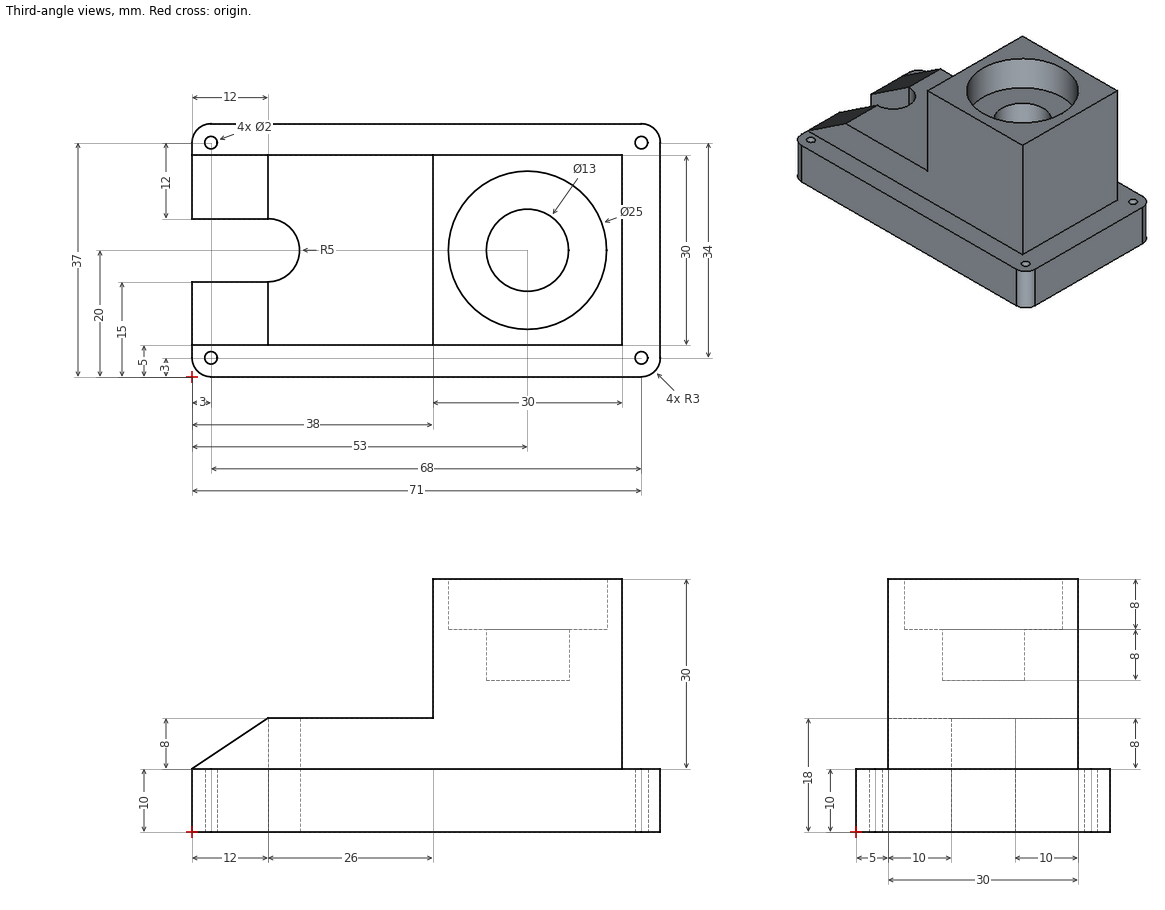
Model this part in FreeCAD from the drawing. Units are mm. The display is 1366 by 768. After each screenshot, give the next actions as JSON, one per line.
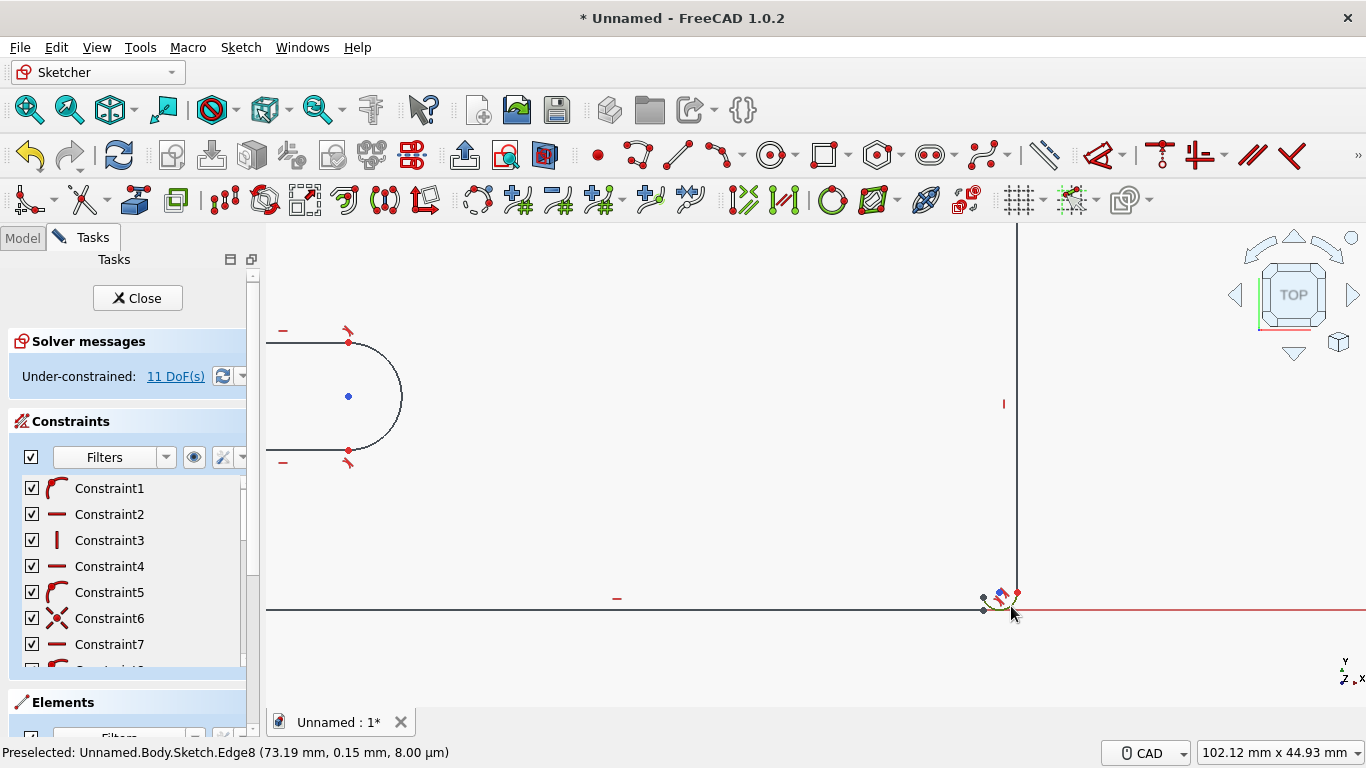
{"action": "scroll", "coordinate": [1013, 608], "scroll_direction": "down", "scroll_amount": 2}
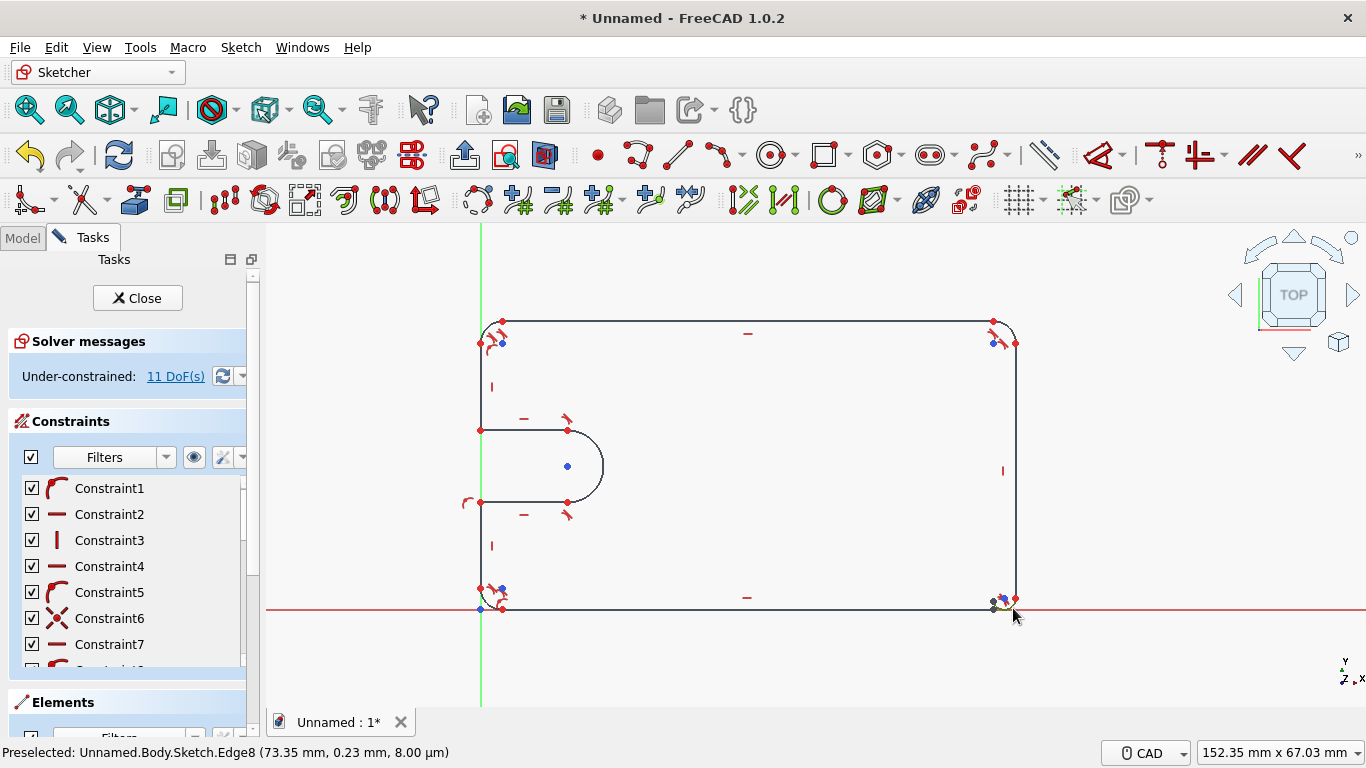
{"action": "scroll", "coordinate": [1013, 334], "scroll_direction": "up", "scroll_amount": 2}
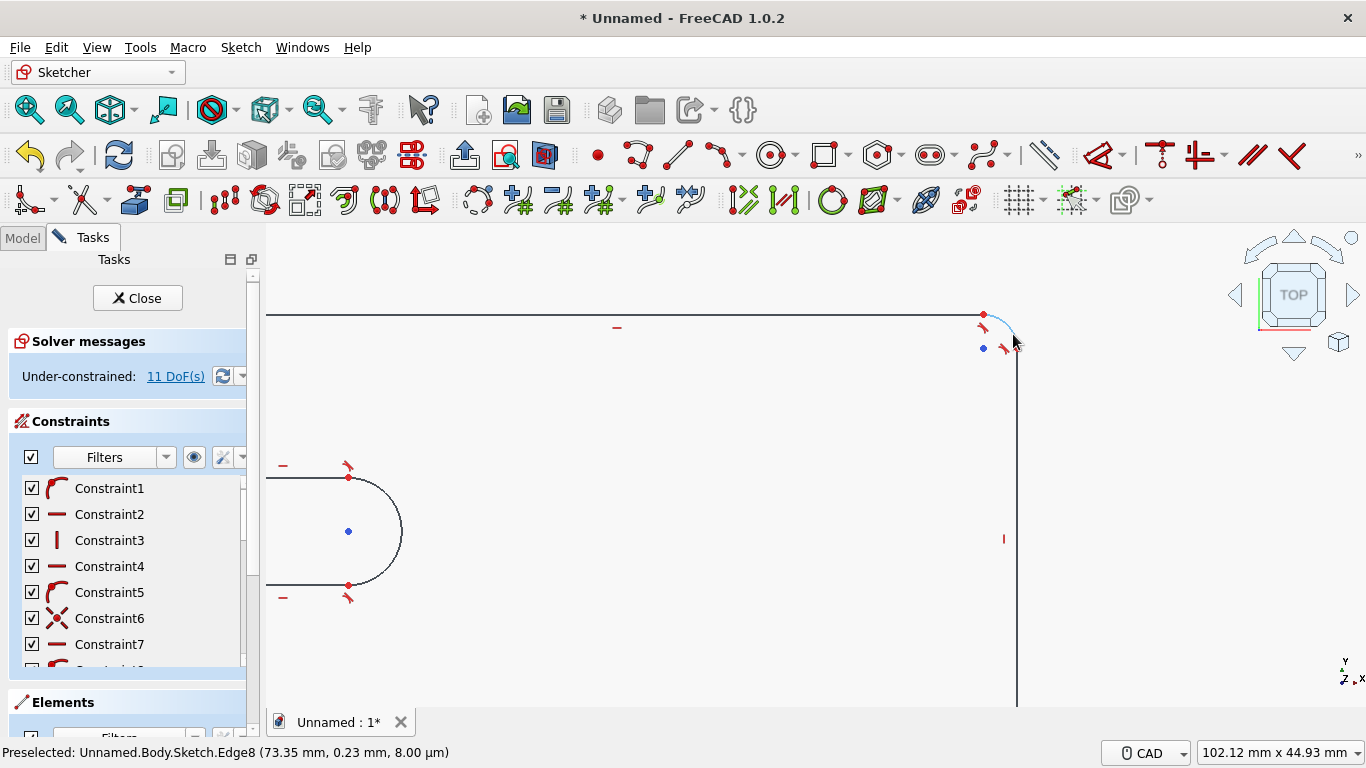
{"action": "left_click", "coordinate": [1013, 333]}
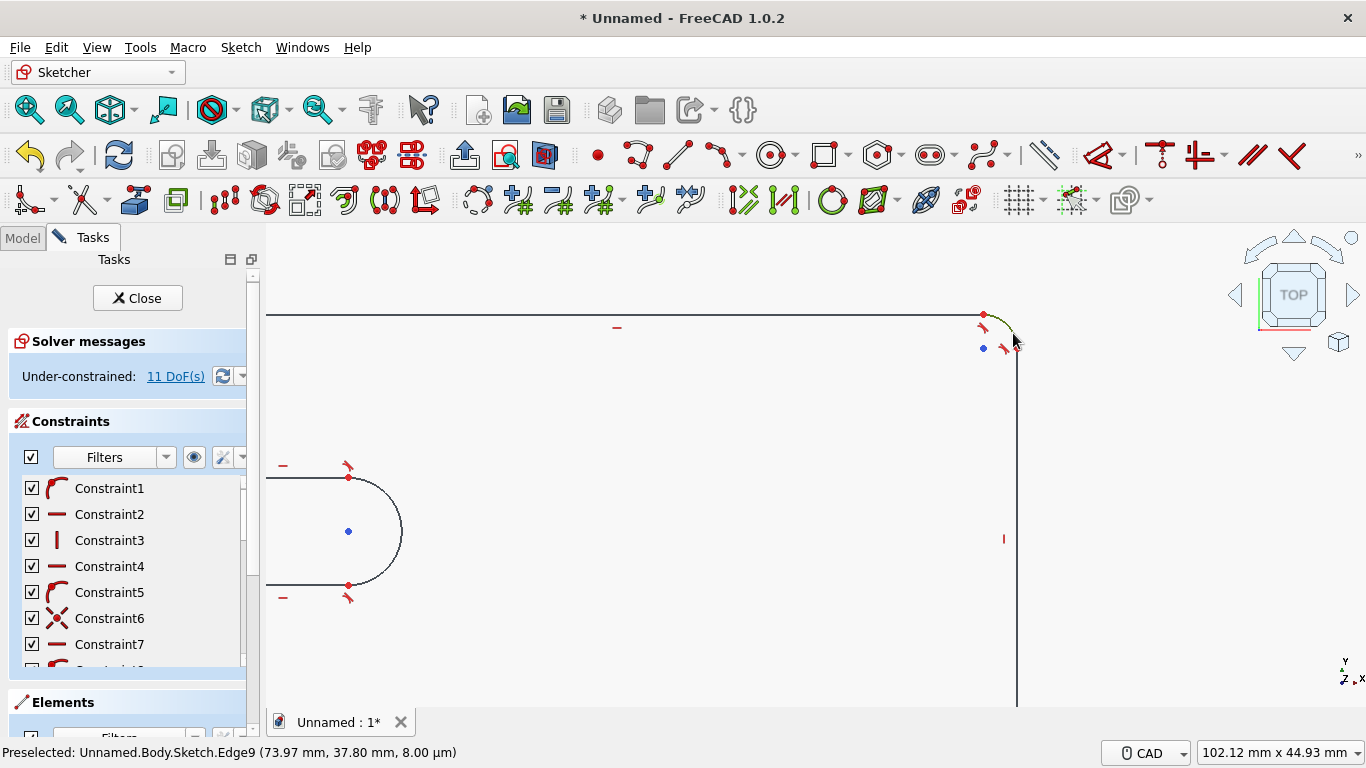
{"action": "scroll", "coordinate": [1013, 333], "scroll_direction": "down", "scroll_amount": 2}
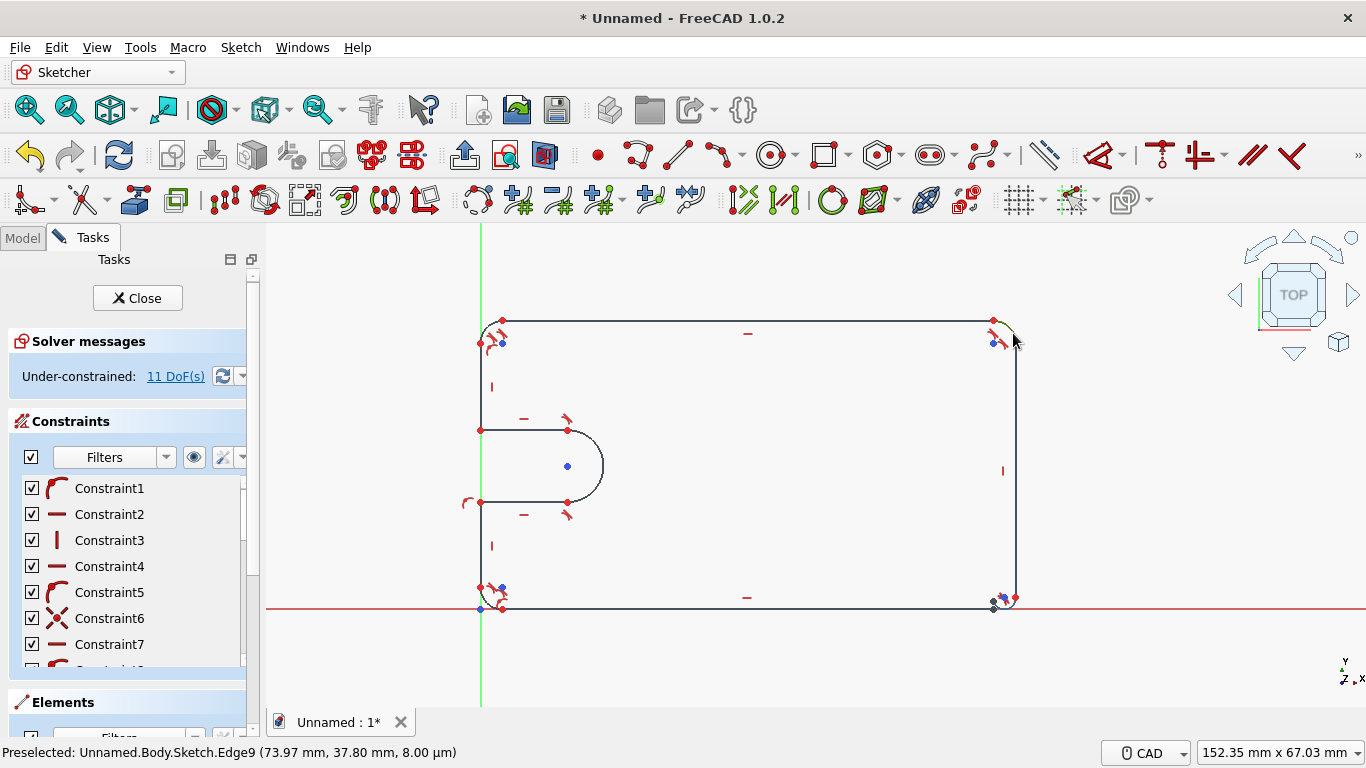
{"action": "scroll", "coordinate": [493, 323], "scroll_direction": "up", "scroll_amount": 2}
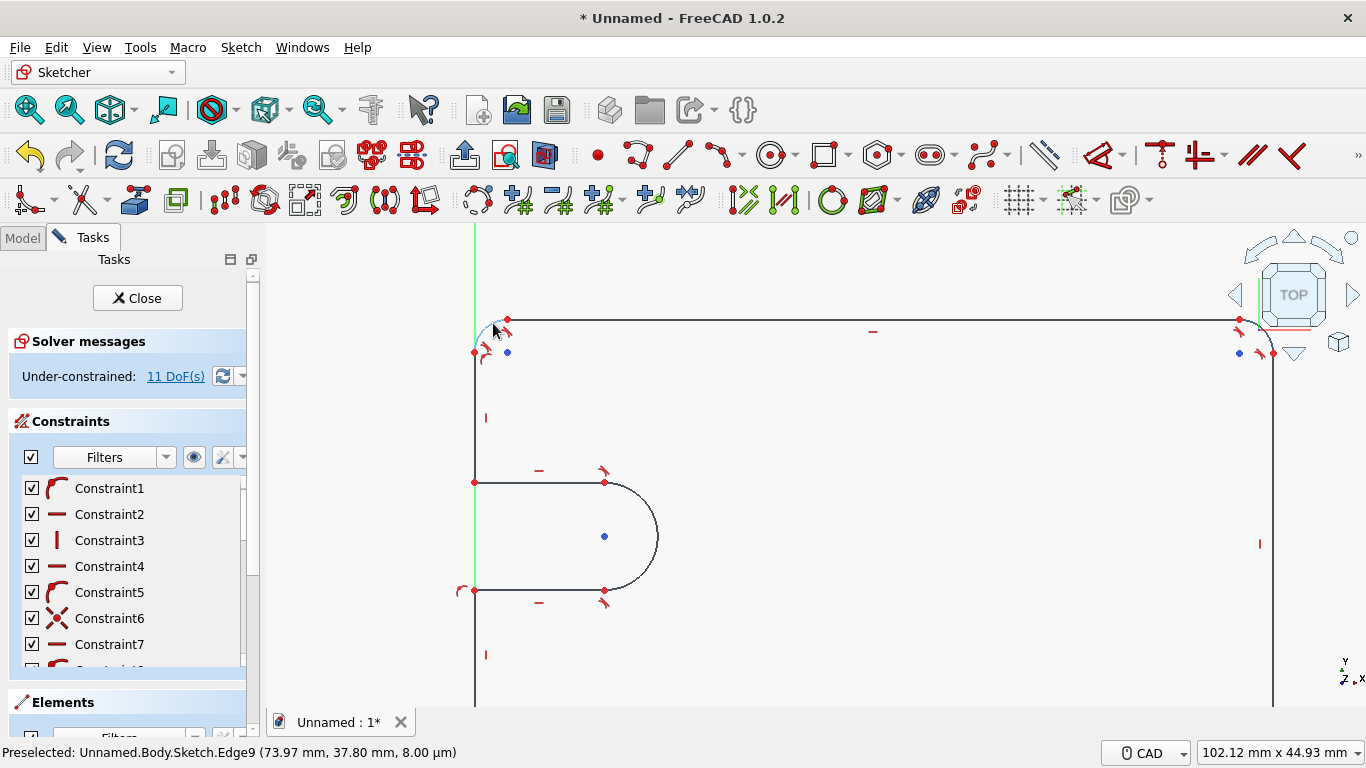
{"action": "left_click", "coordinate": [493, 323]}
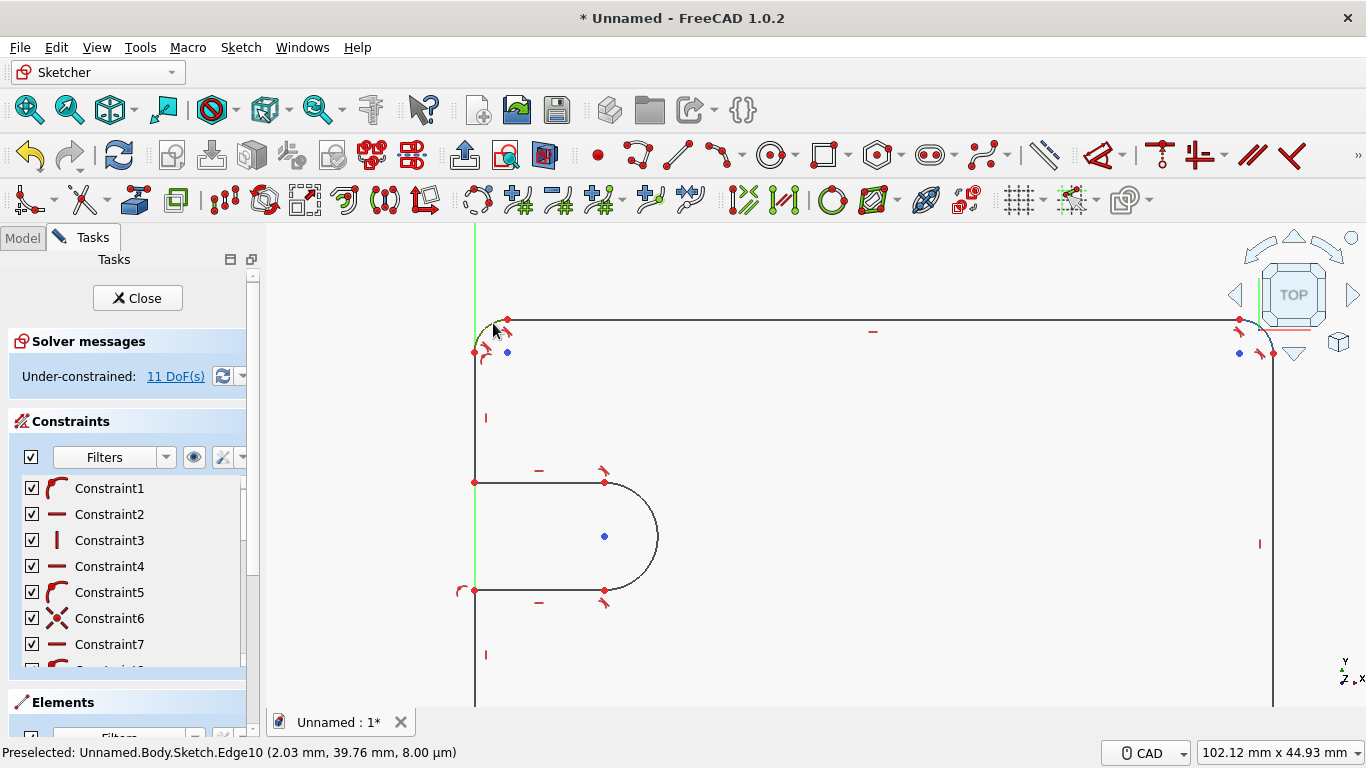
{"action": "scroll", "coordinate": [492, 323], "scroll_direction": "down", "scroll_amount": 2}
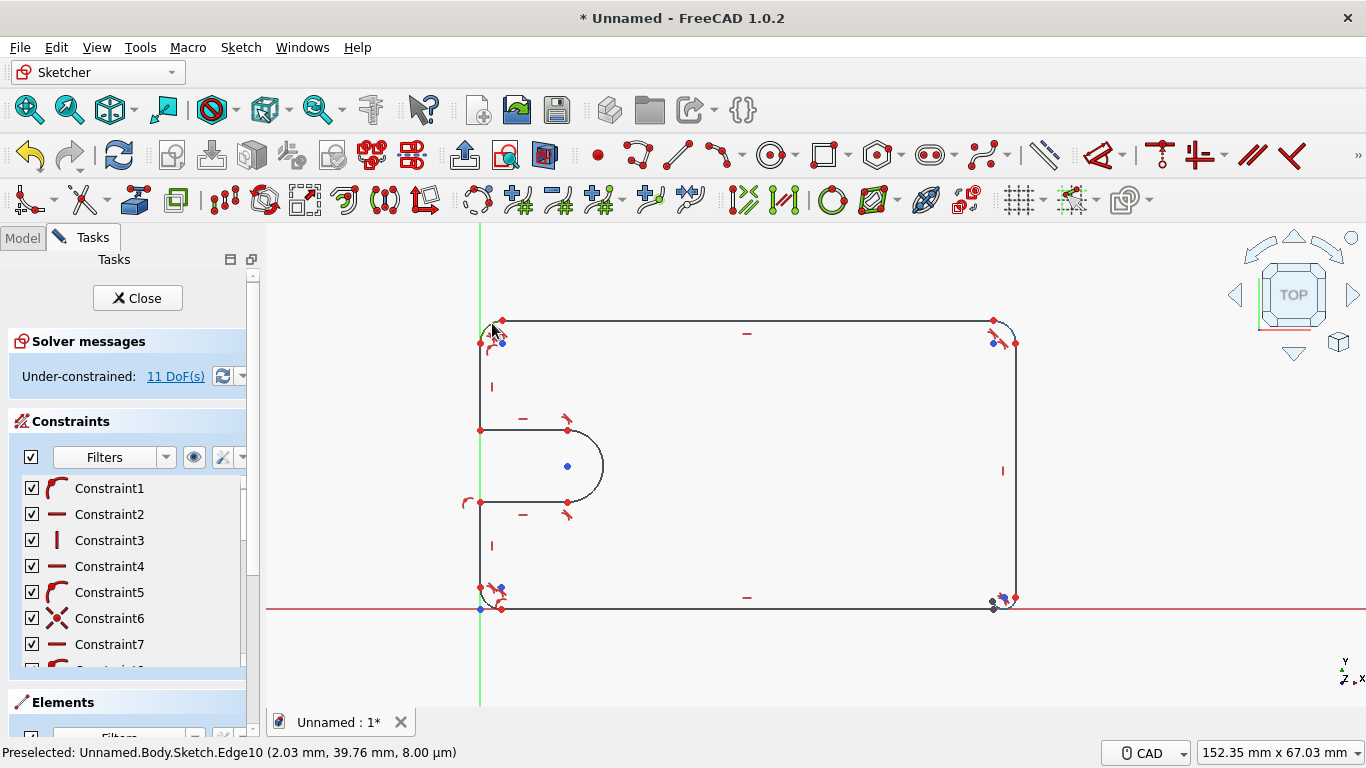
{"action": "scroll", "coordinate": [483, 598], "scroll_direction": "up", "scroll_amount": 2}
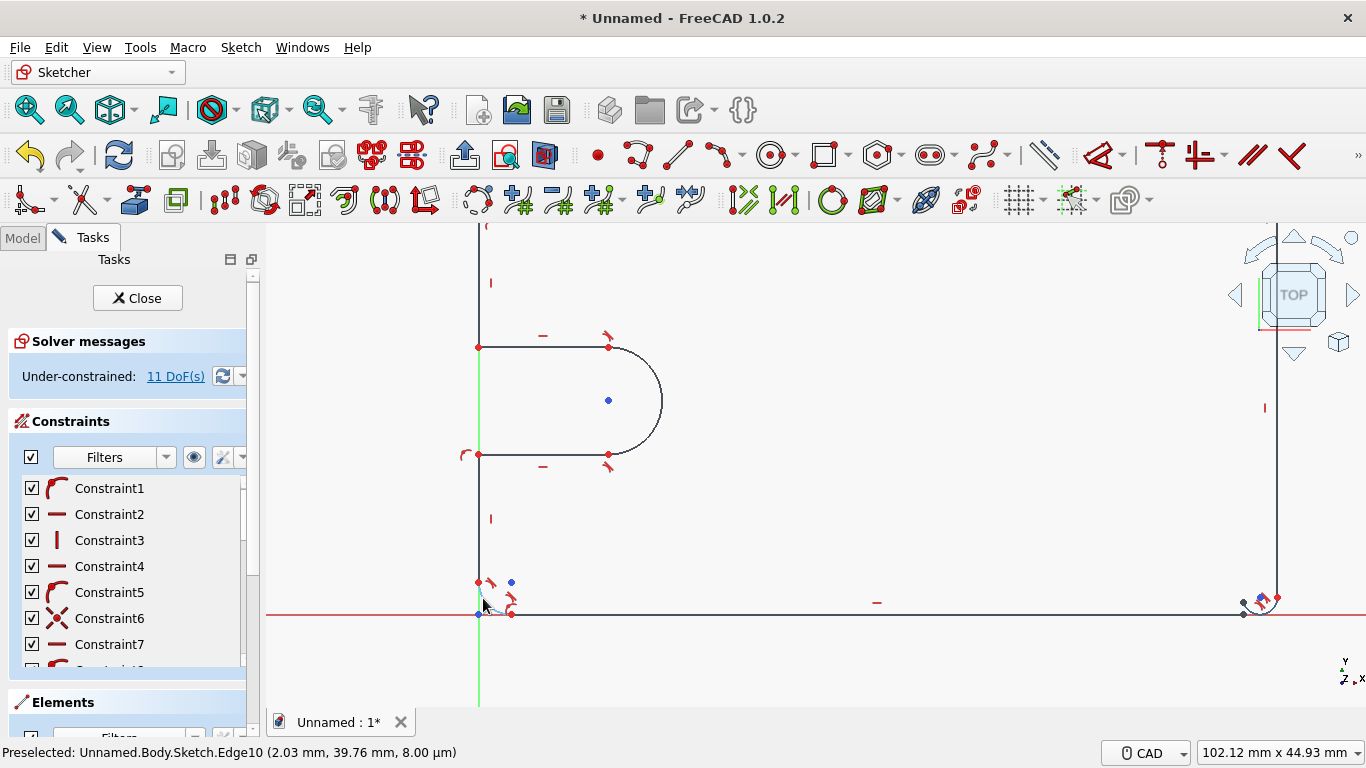
{"action": "left_click", "coordinate": [482, 597]}